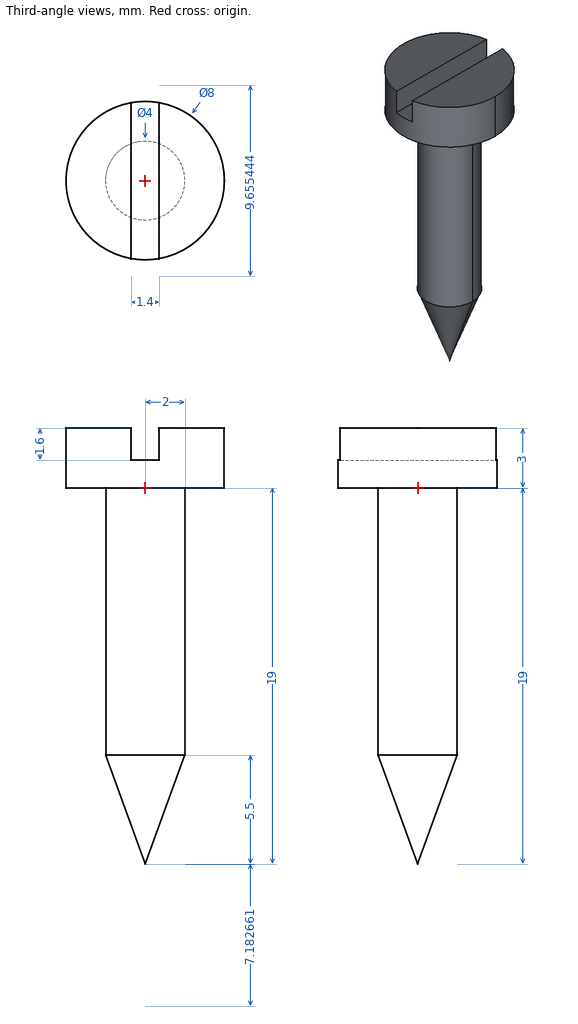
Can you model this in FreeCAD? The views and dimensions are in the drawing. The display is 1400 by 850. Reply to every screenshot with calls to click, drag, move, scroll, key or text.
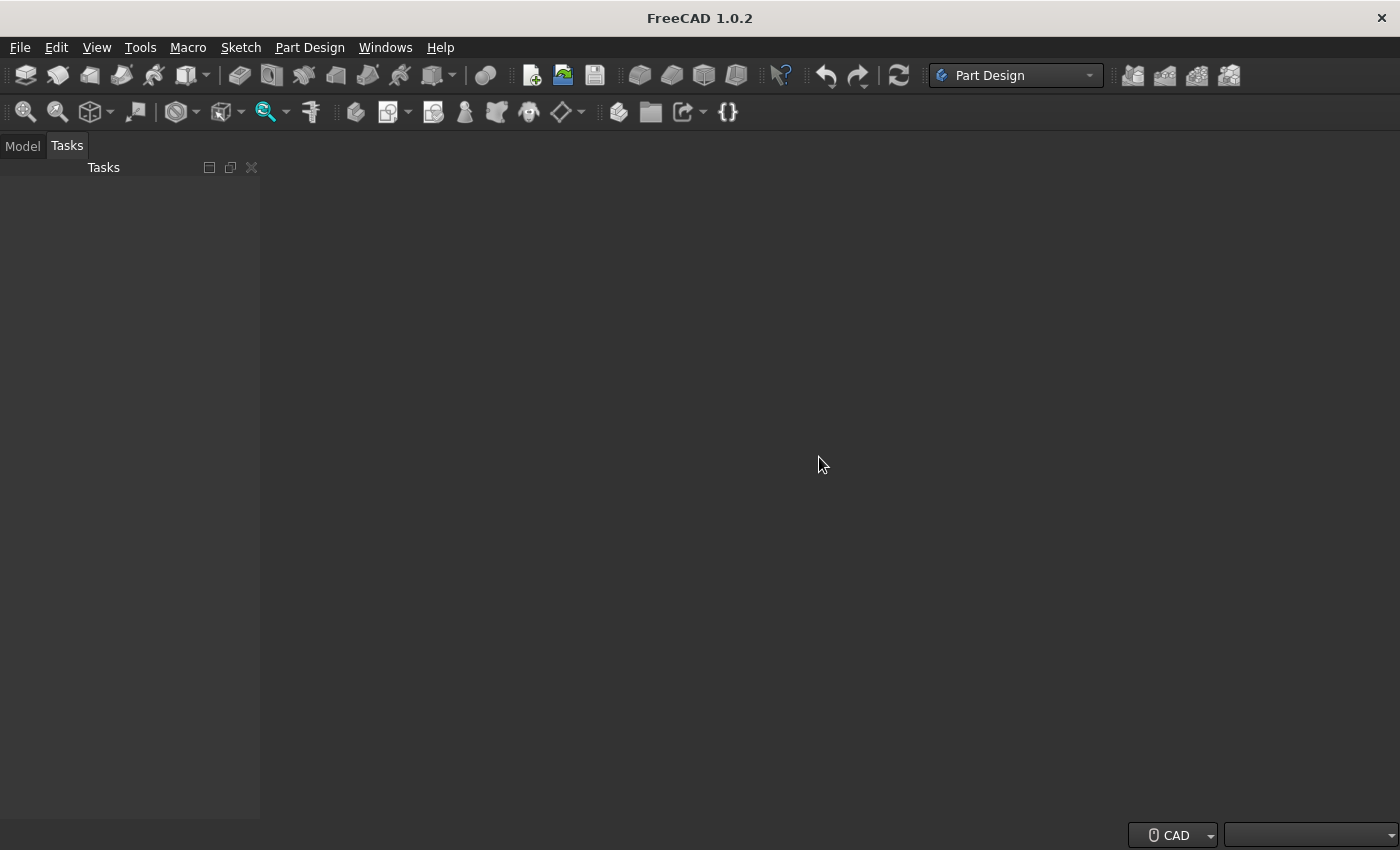
key(ctrl+n)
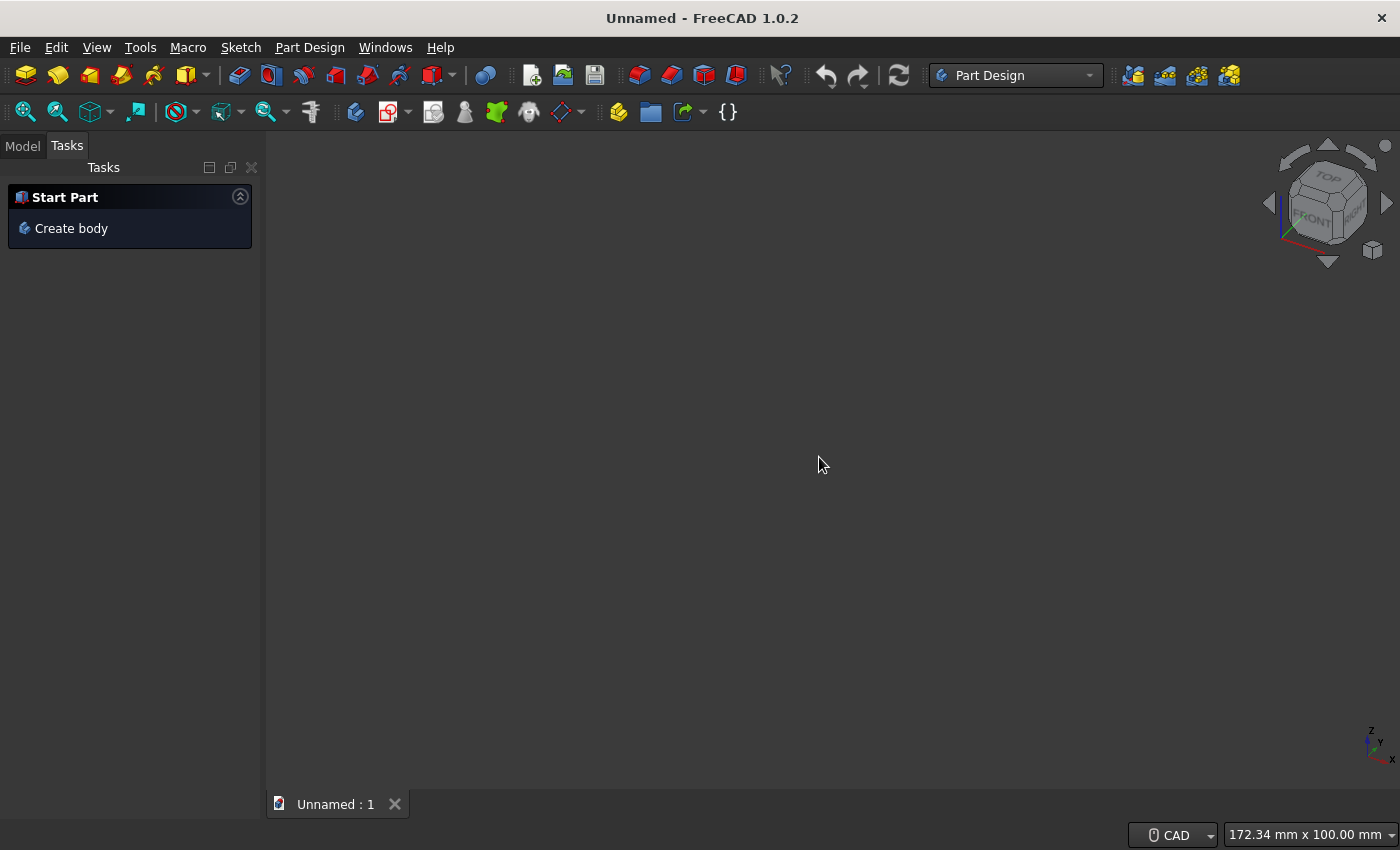
click(388, 112)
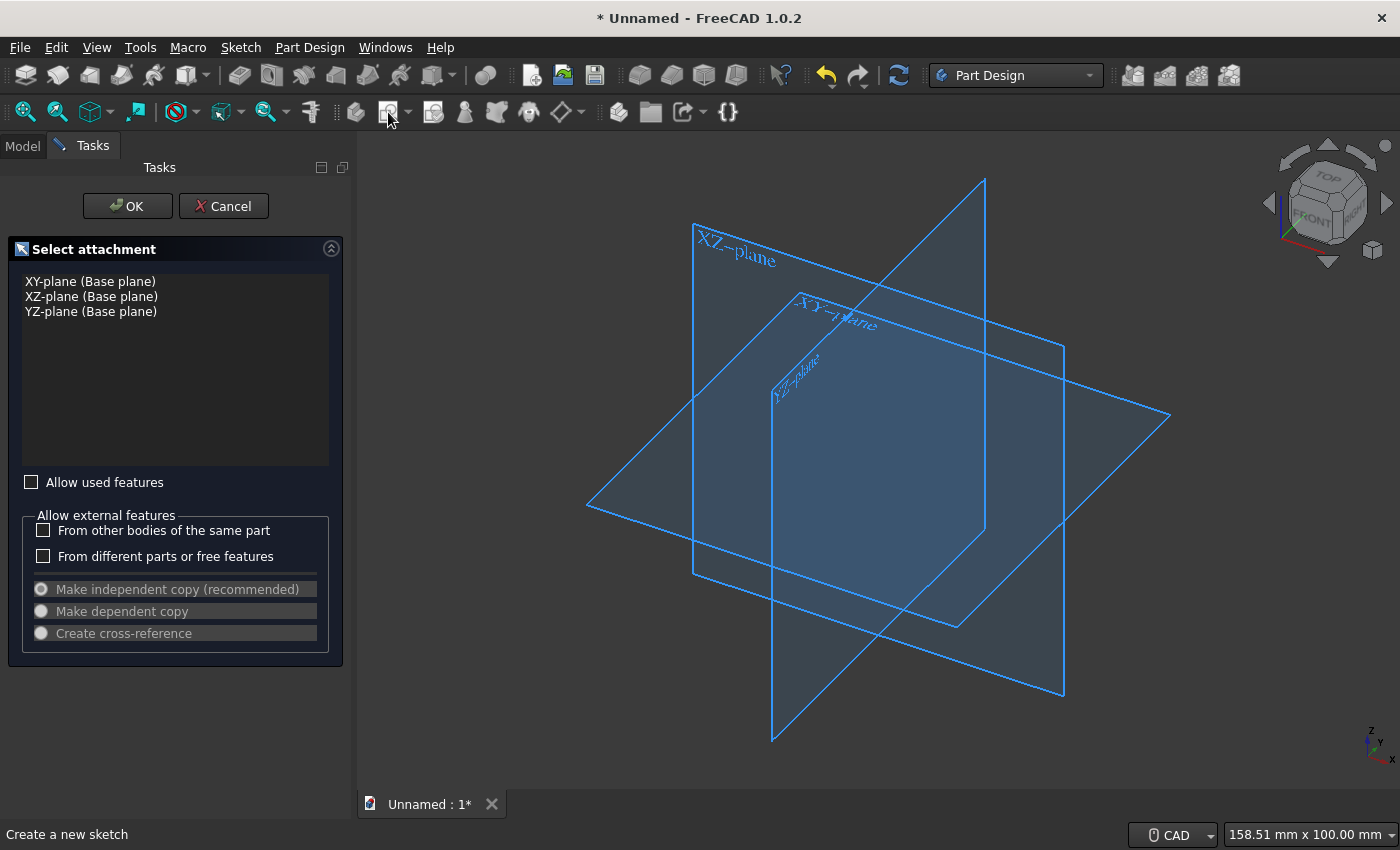
click(82, 282)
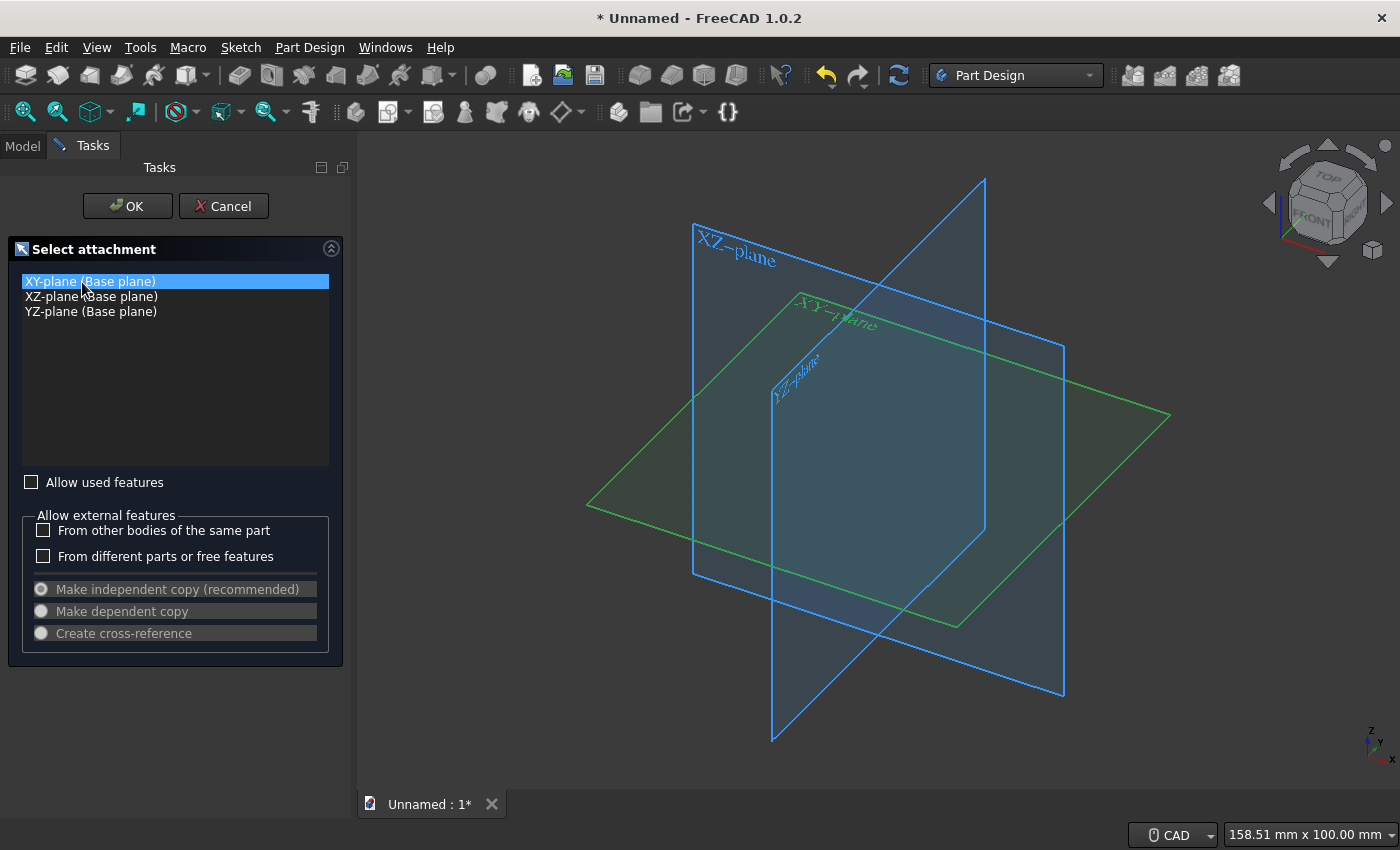
click(128, 206)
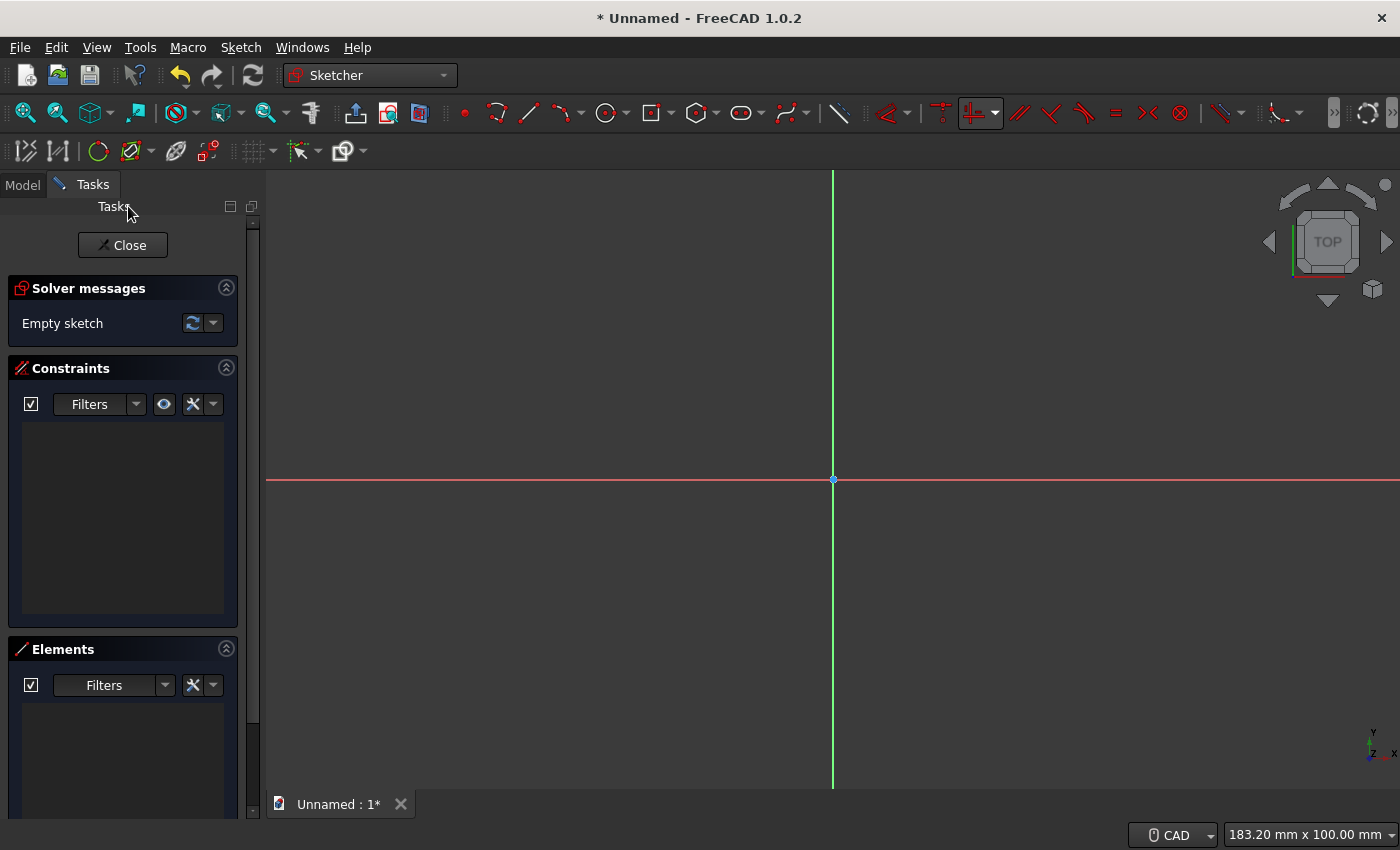
scroll(844, 480, up, 10)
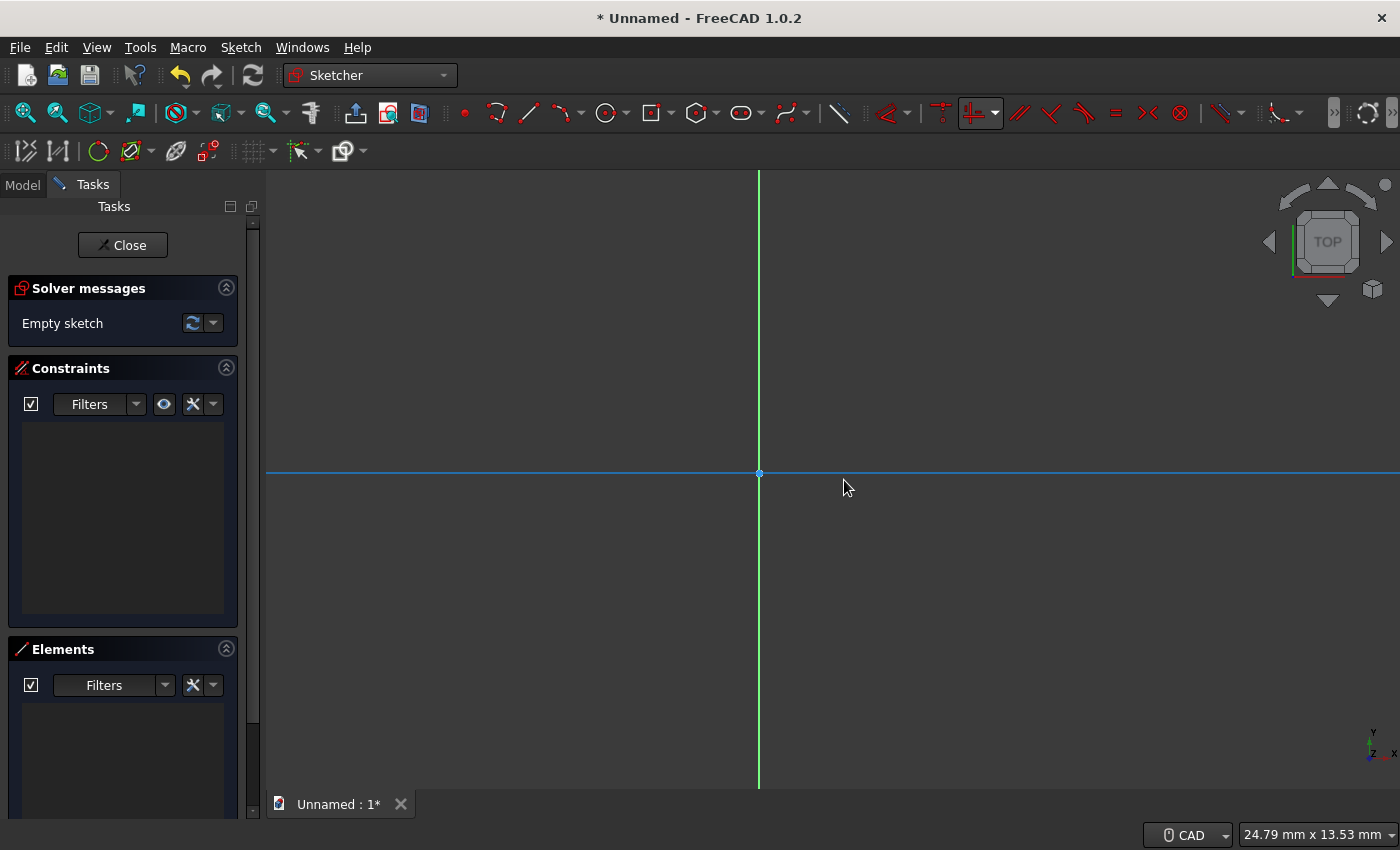
click(606, 114)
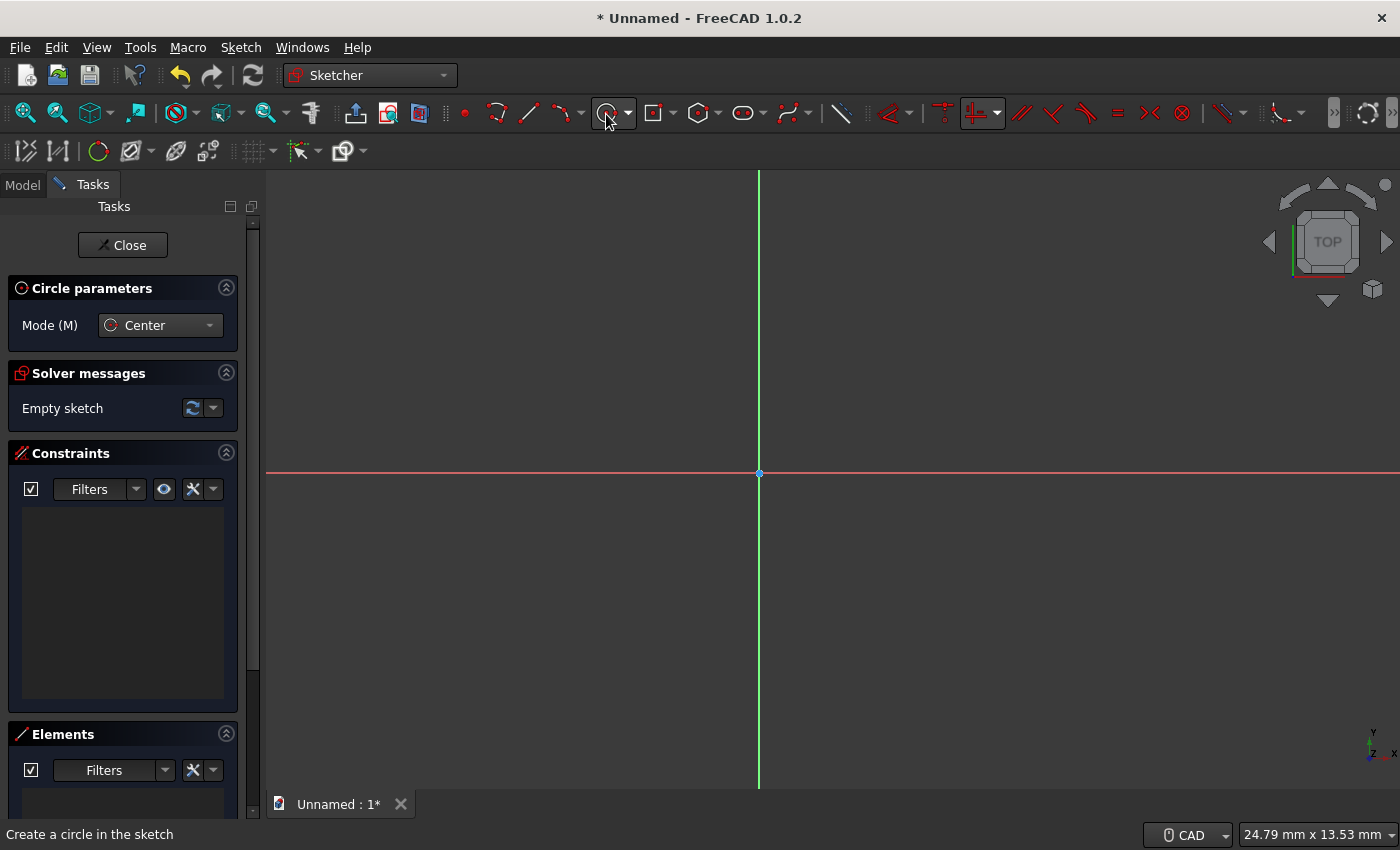
click(759, 473)
move(889, 344)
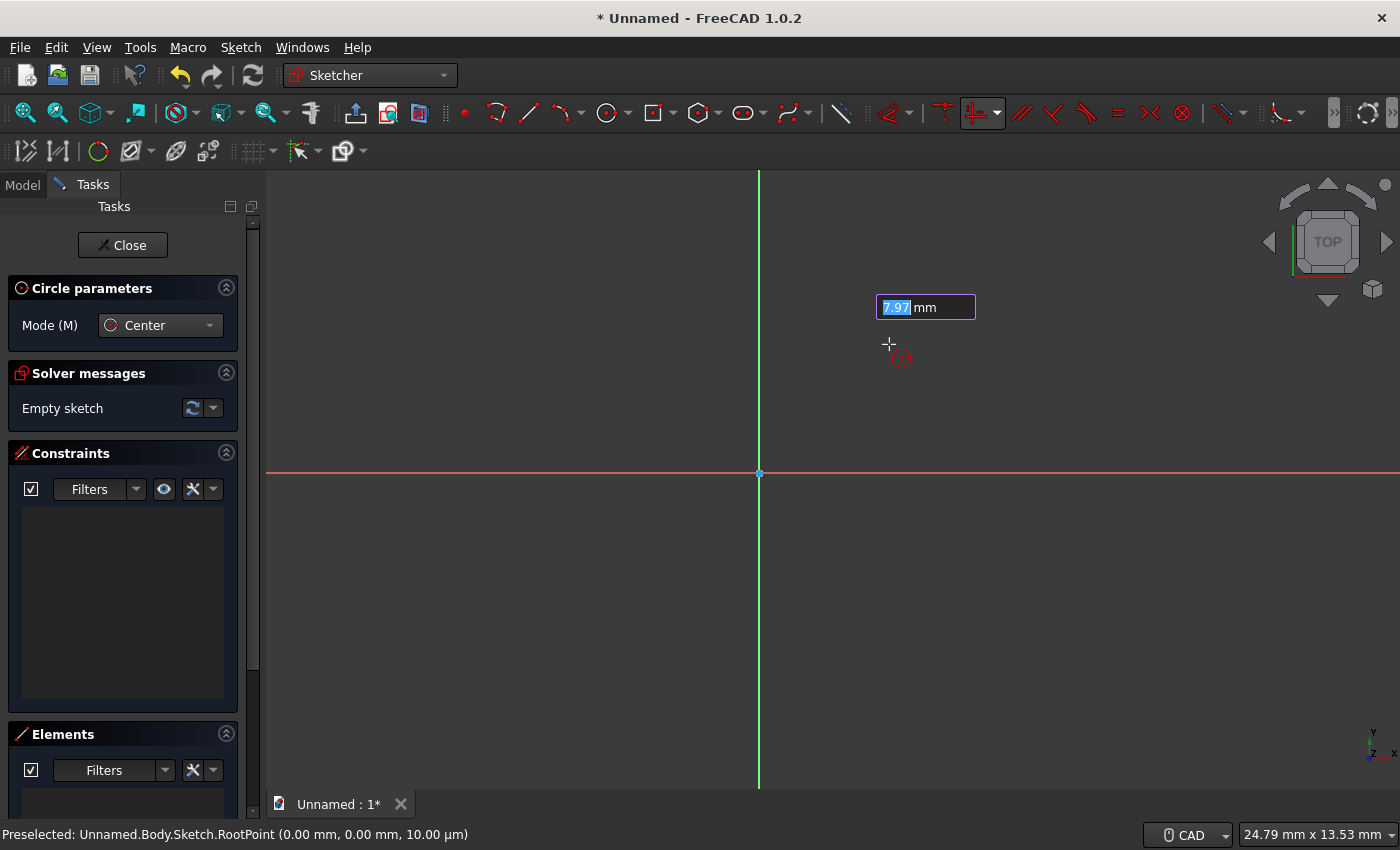
text(8)
key(Return)
key(Escape)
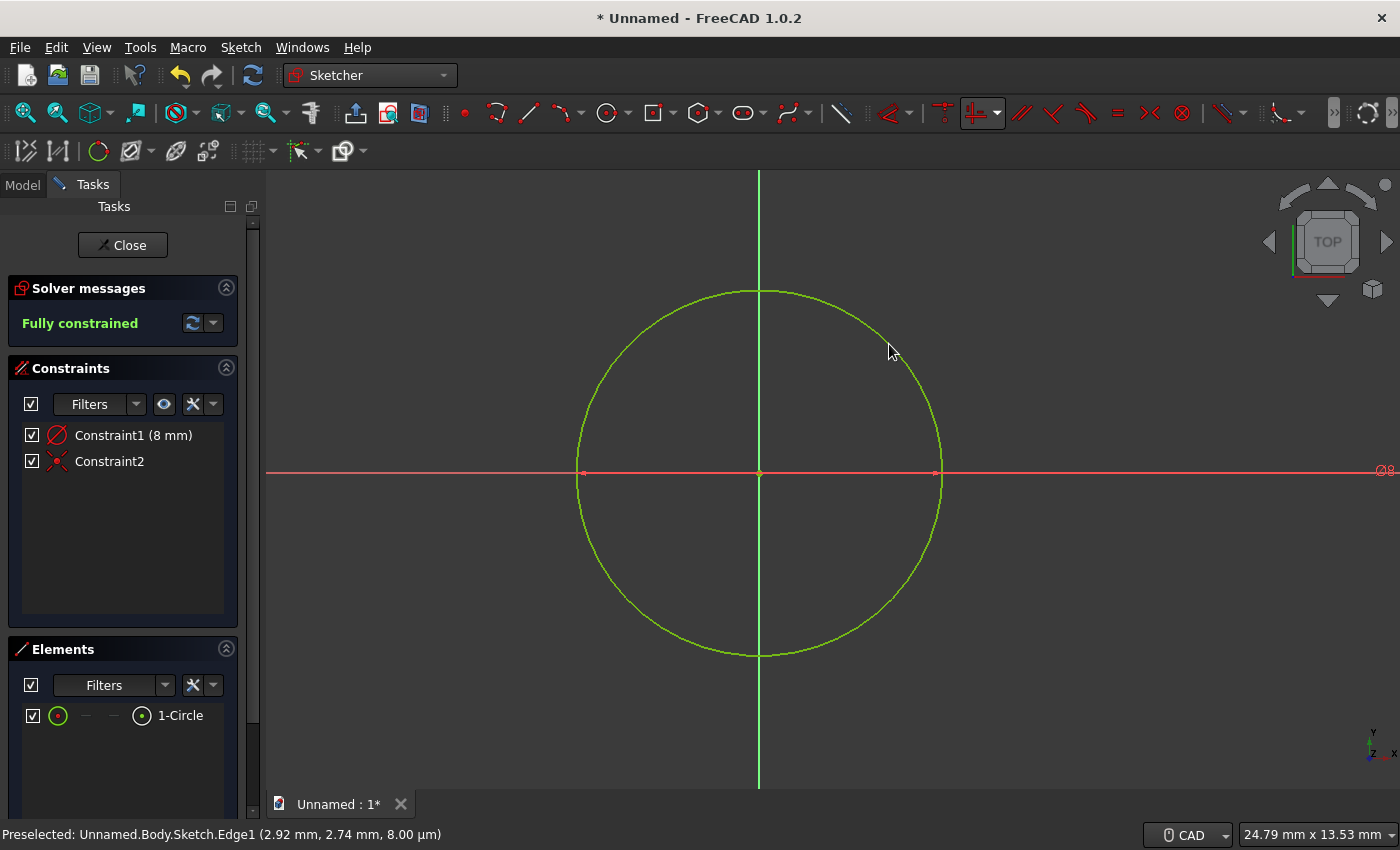
click(123, 245)